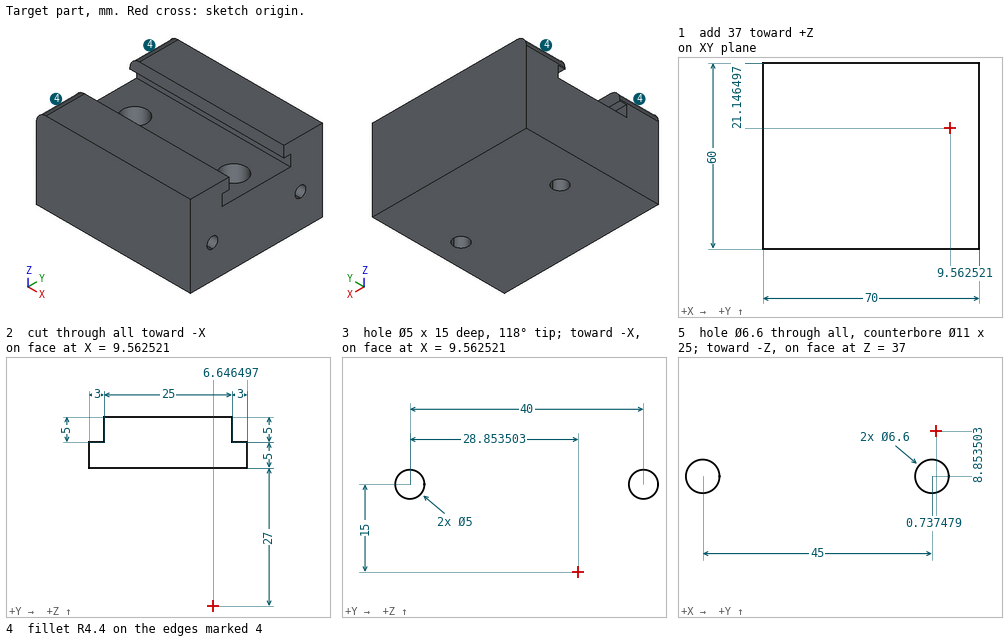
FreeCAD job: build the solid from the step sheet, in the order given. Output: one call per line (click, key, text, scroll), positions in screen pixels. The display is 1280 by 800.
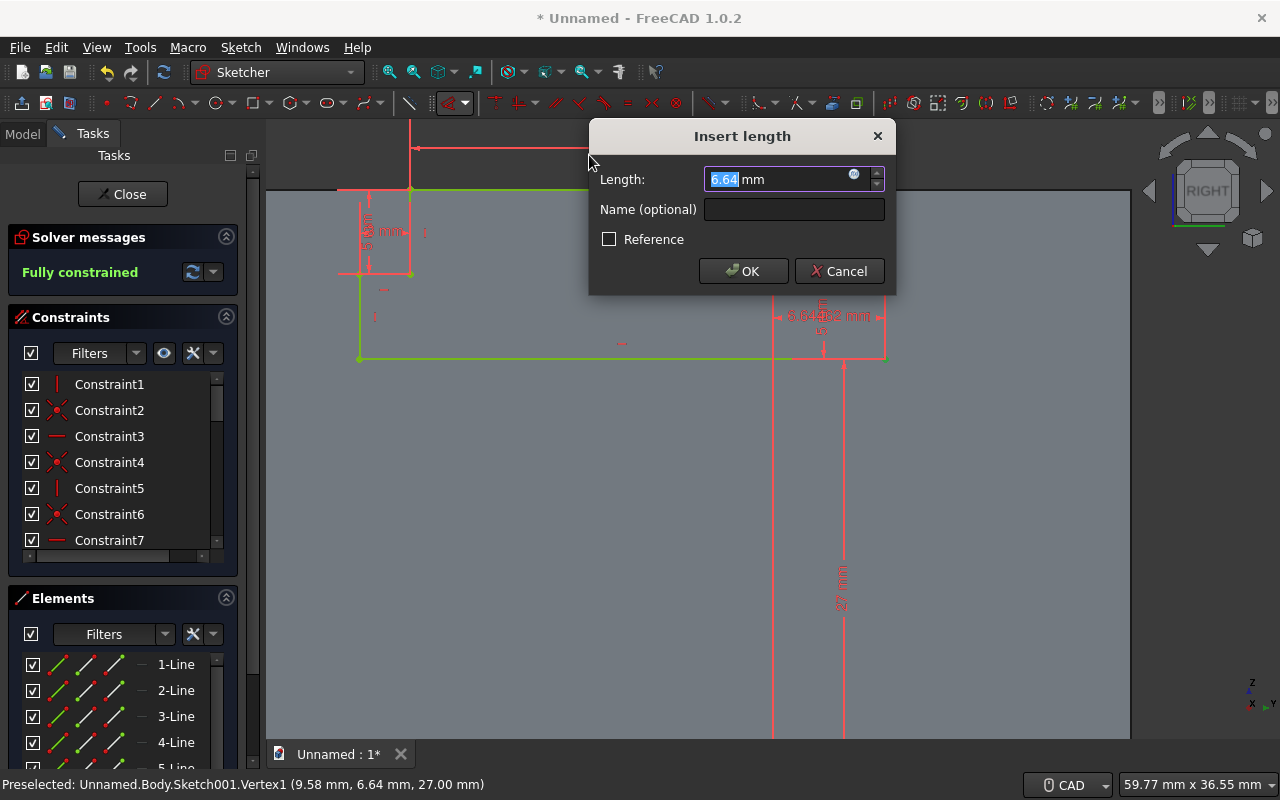
text(6.646497)
key(Return)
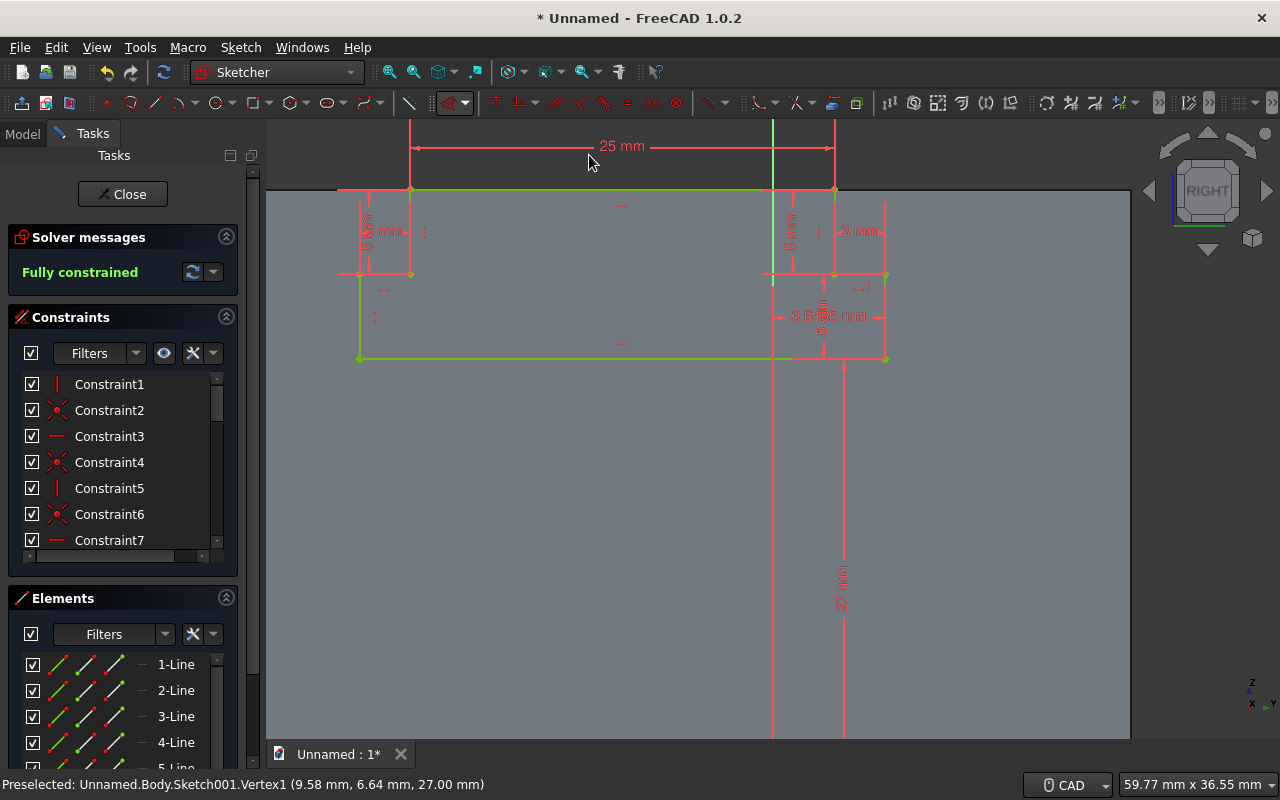
click(123, 194)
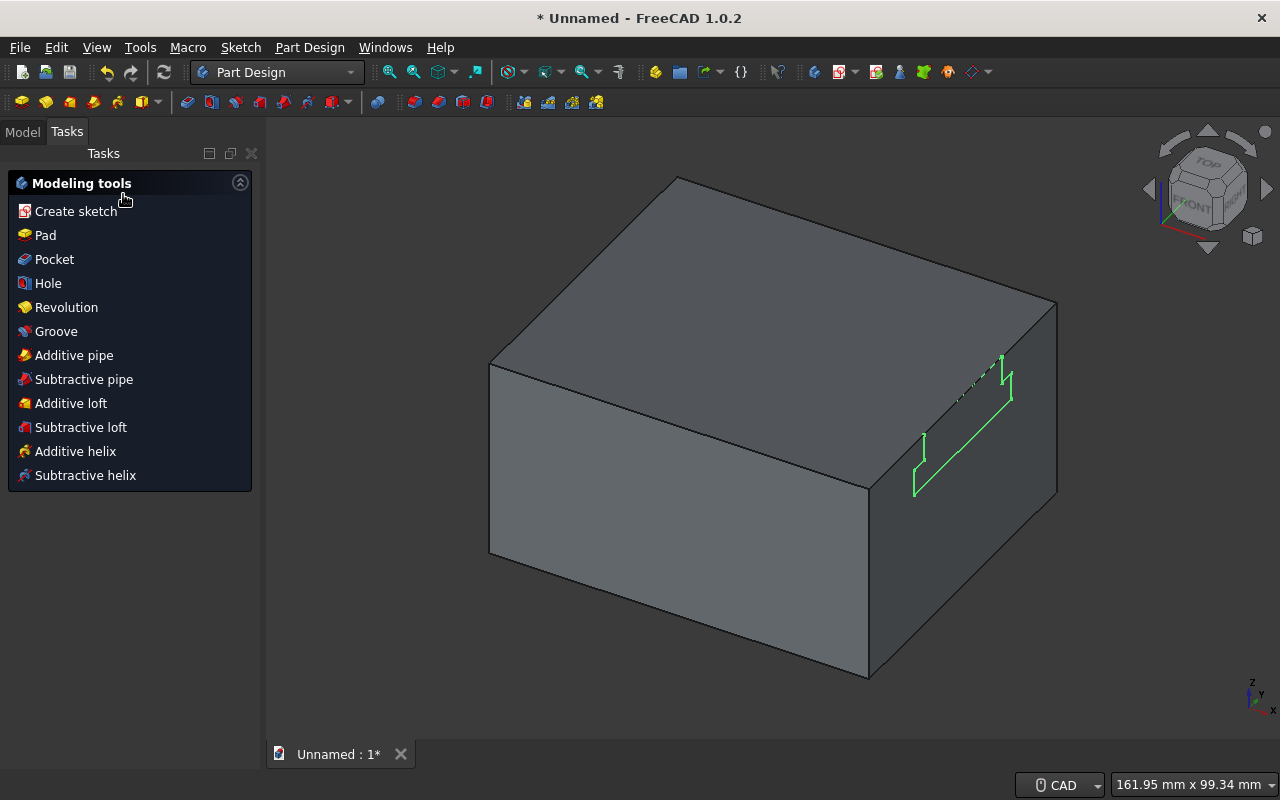
click(188, 102)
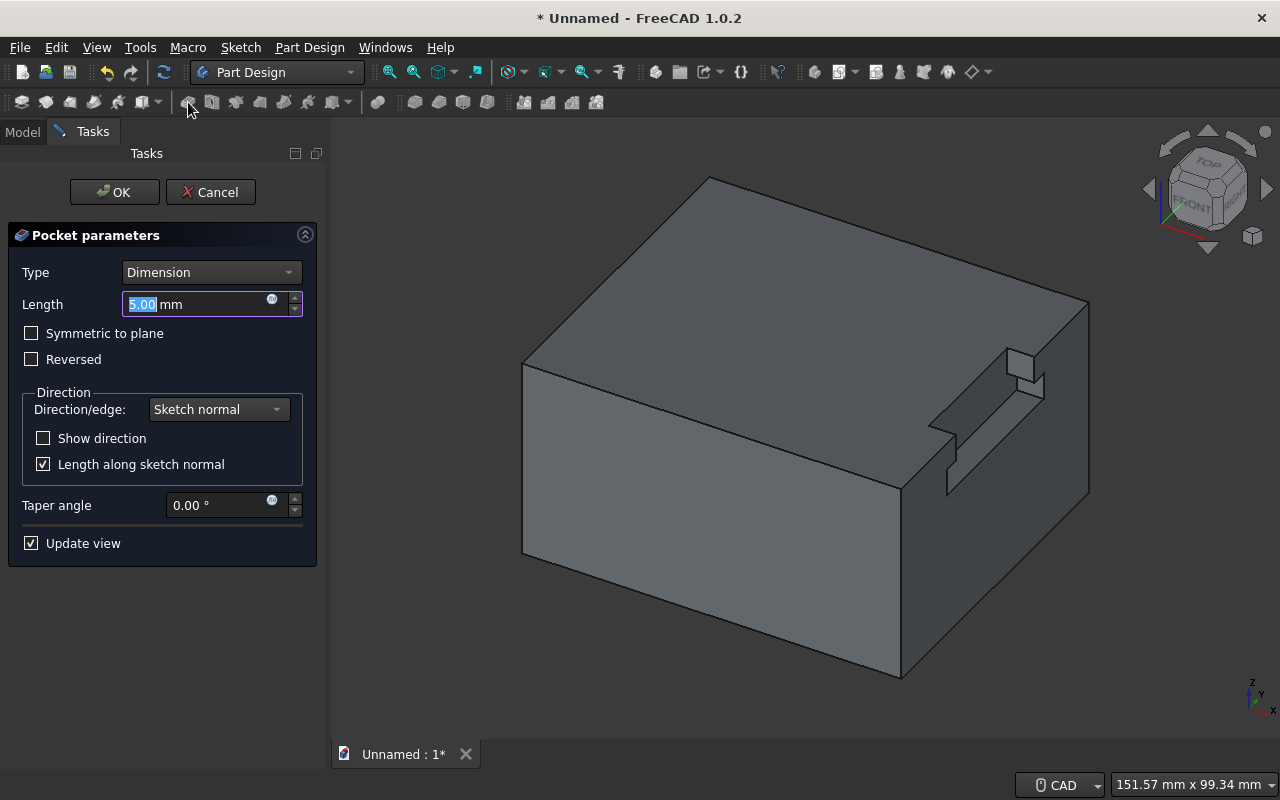
click(212, 272)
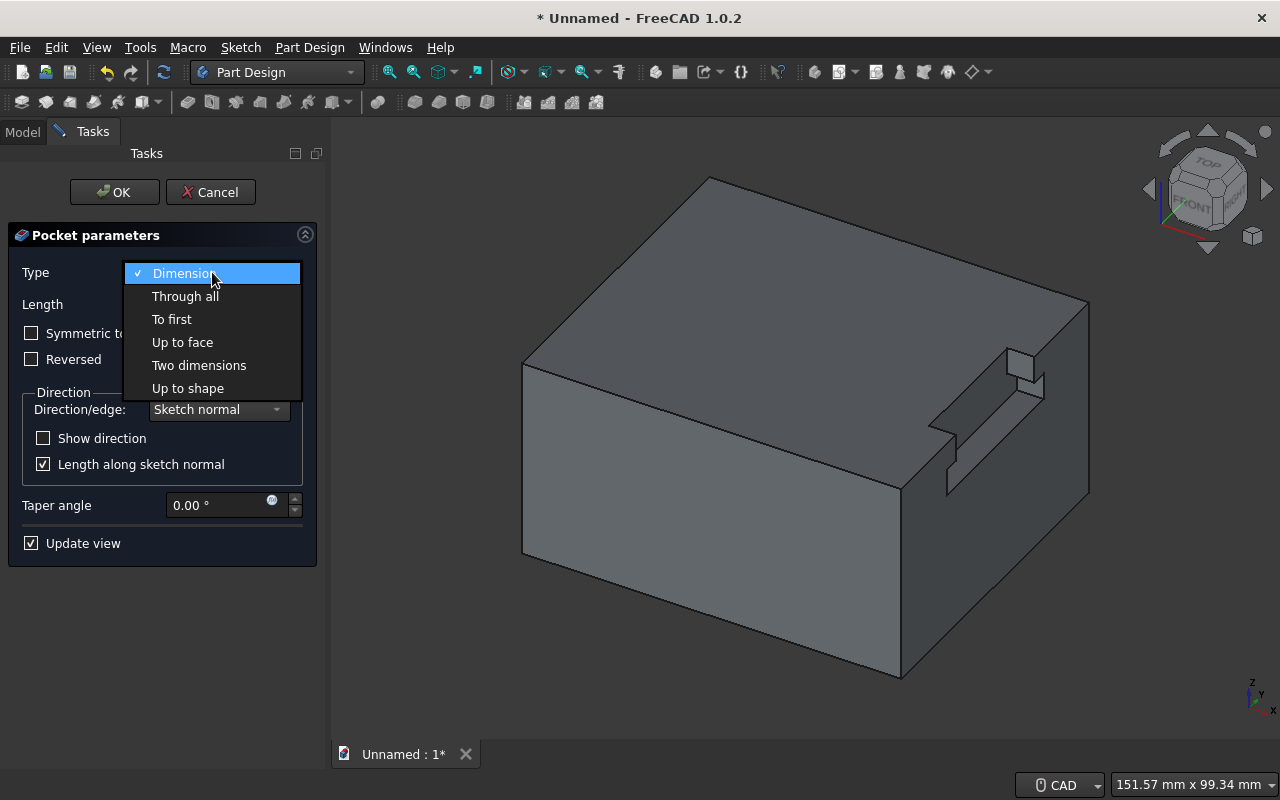
click(212, 296)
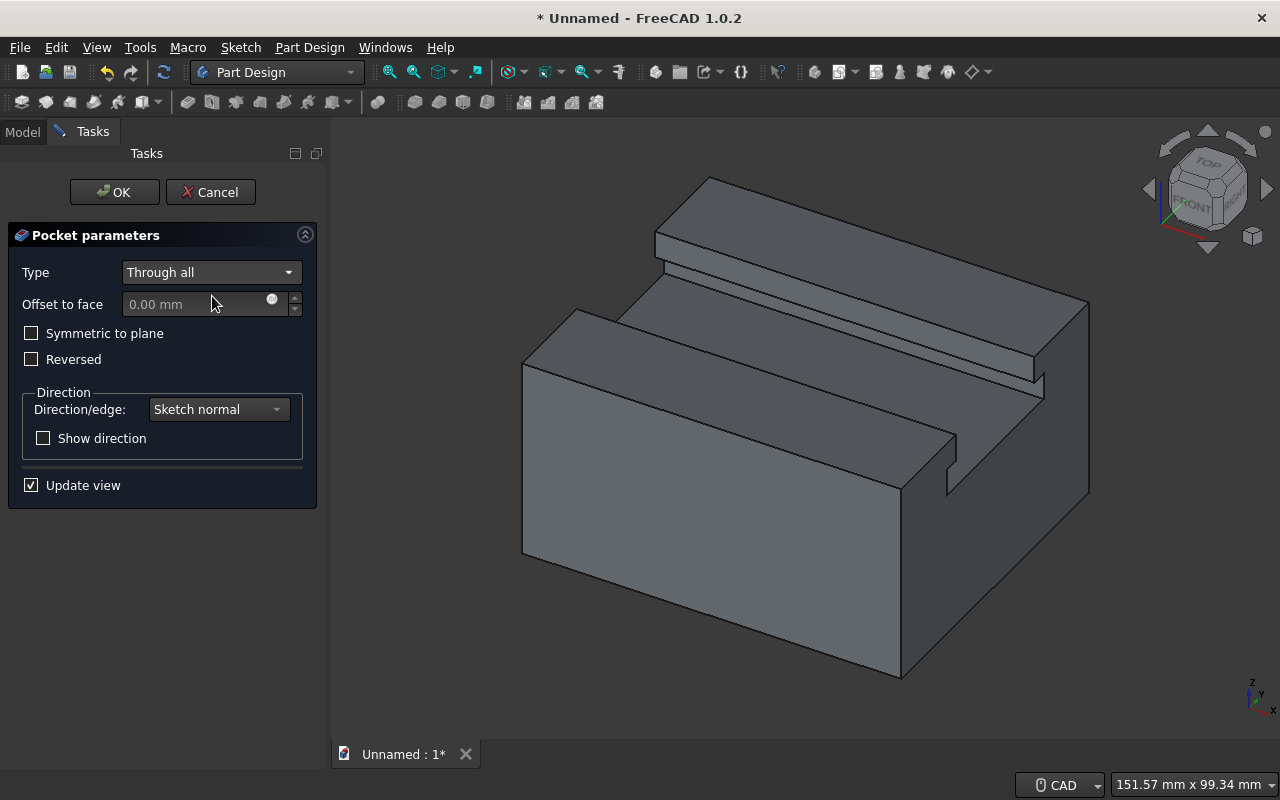
click(115, 192)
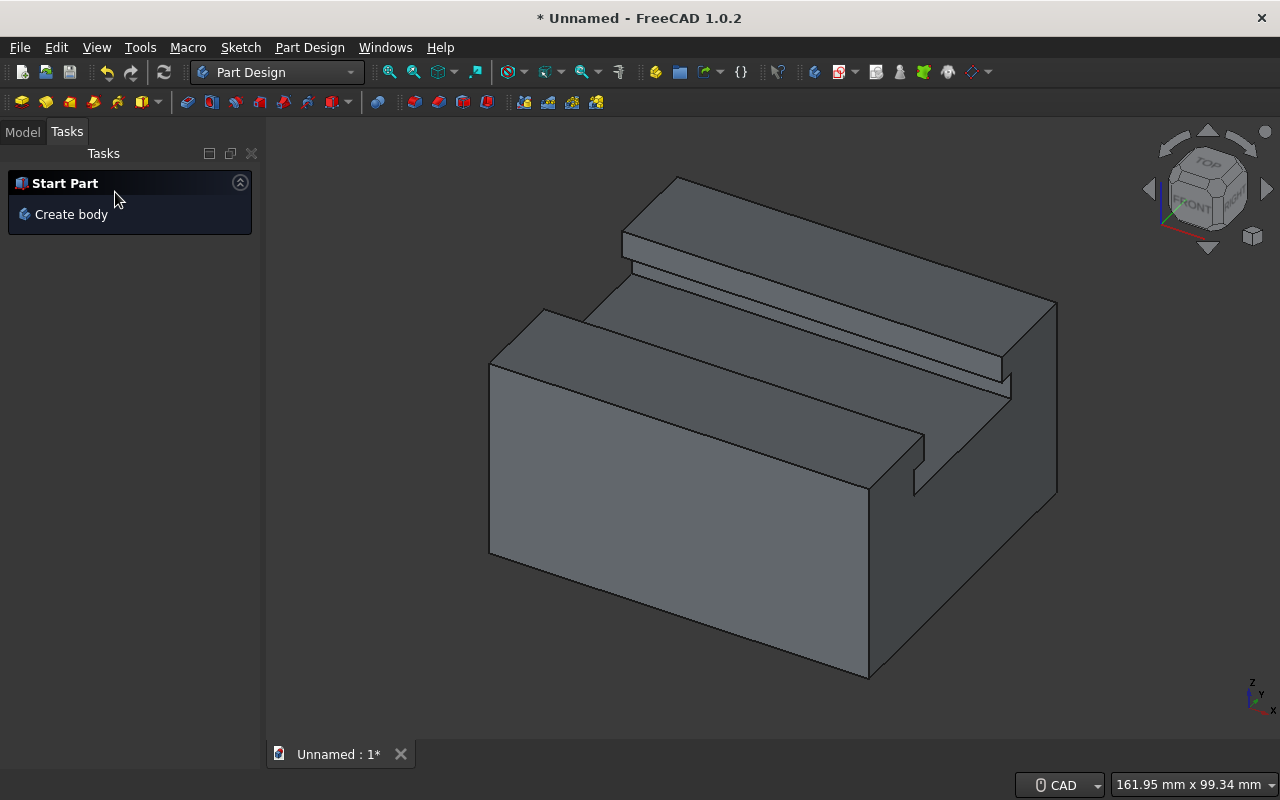
click(990, 490)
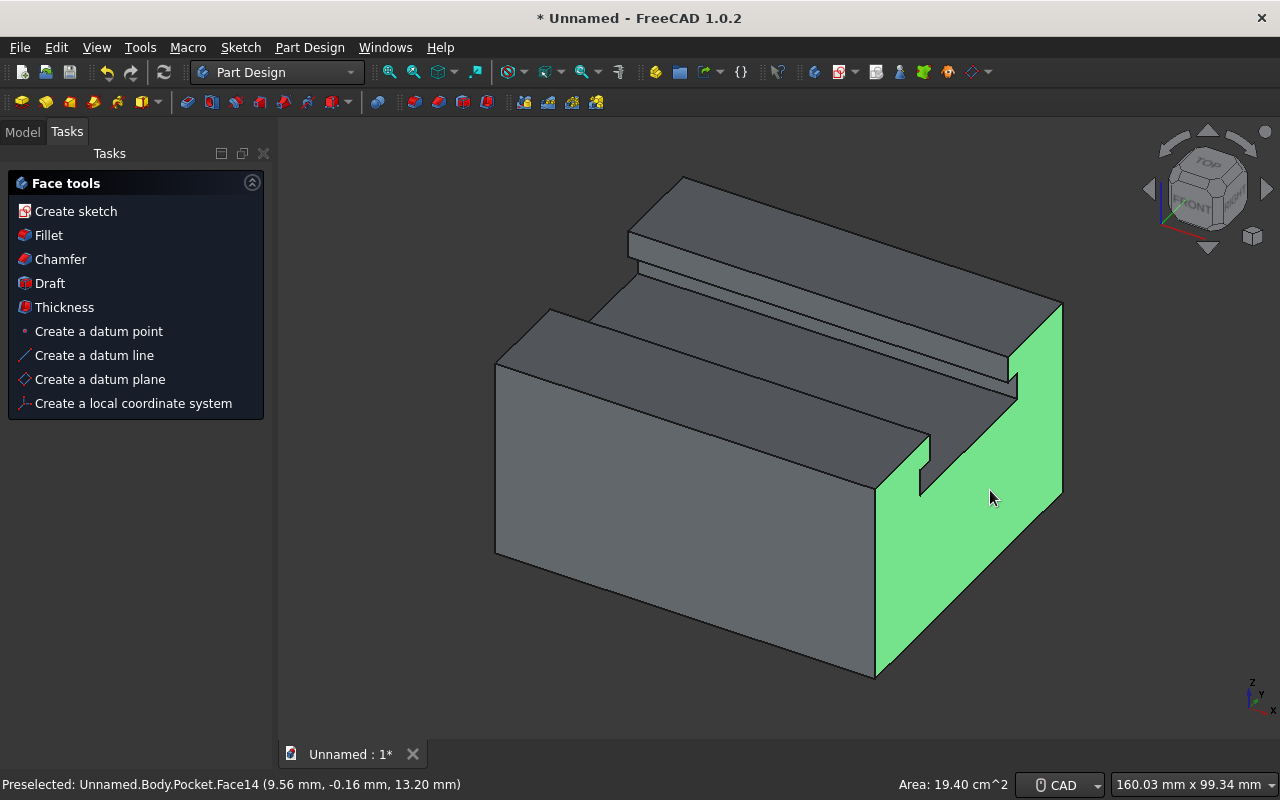
click(840, 72)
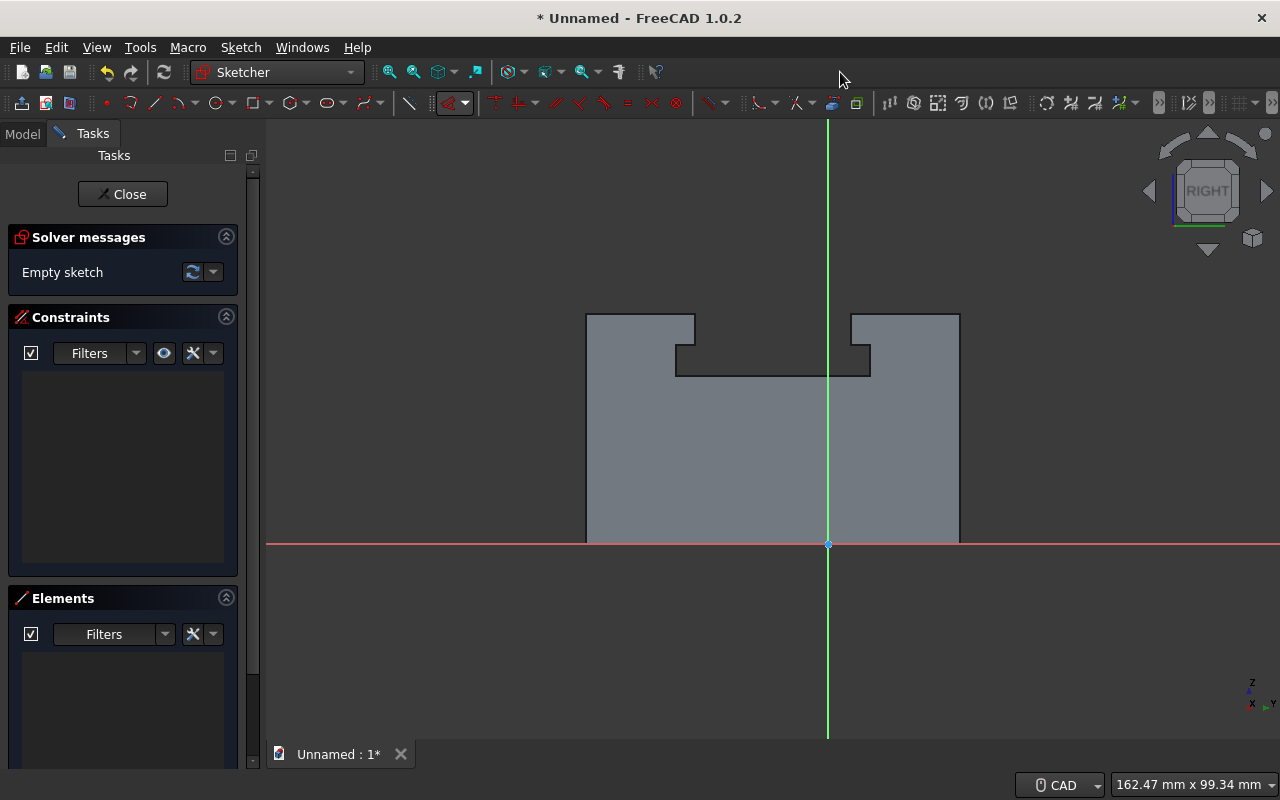
scroll(829, 540, up, 4)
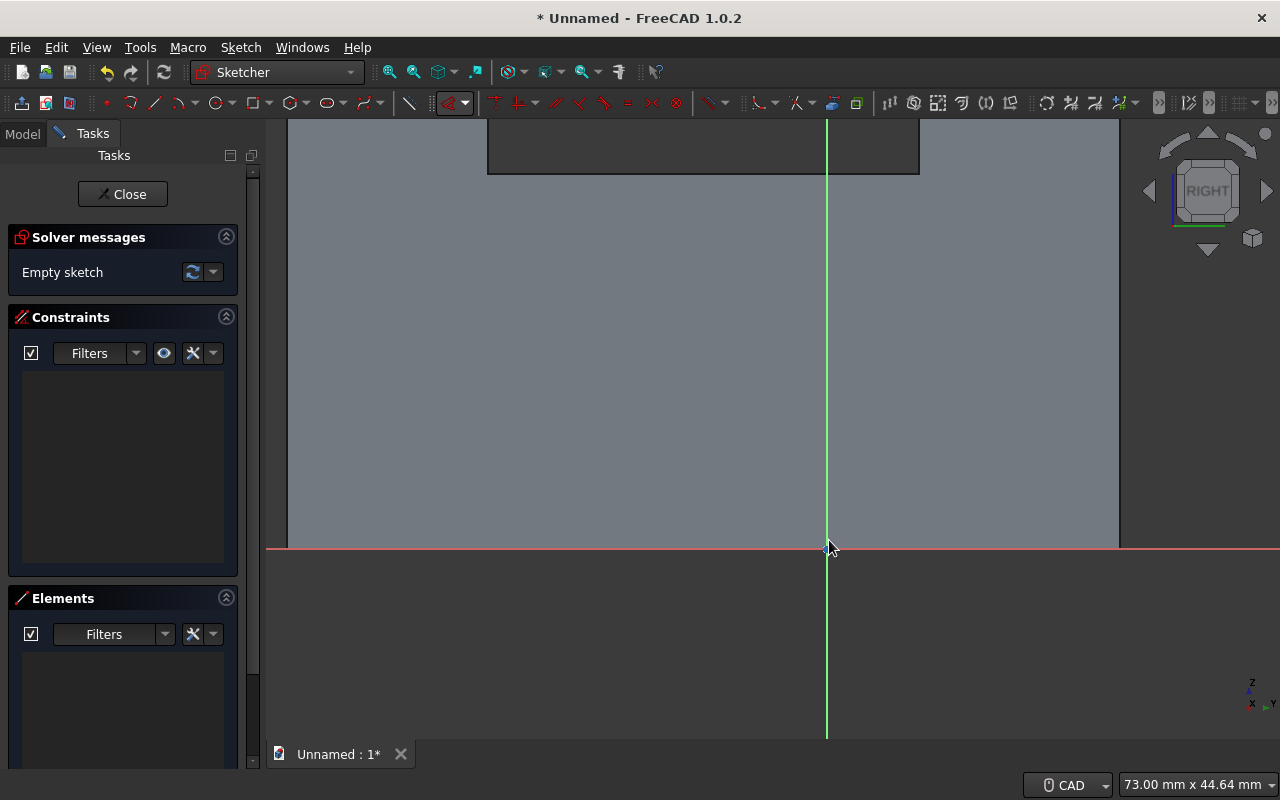
click(216, 104)